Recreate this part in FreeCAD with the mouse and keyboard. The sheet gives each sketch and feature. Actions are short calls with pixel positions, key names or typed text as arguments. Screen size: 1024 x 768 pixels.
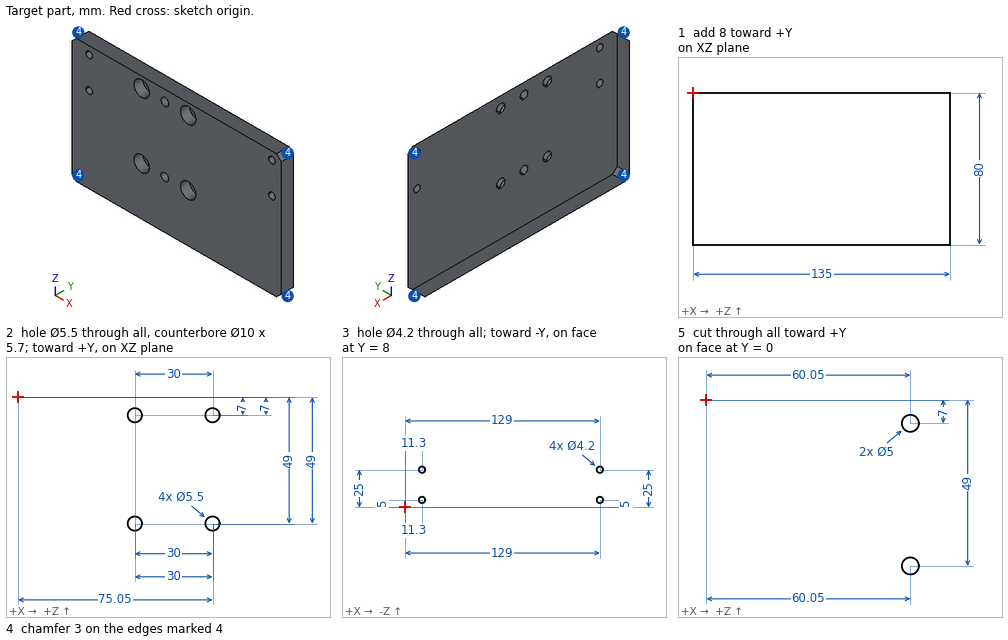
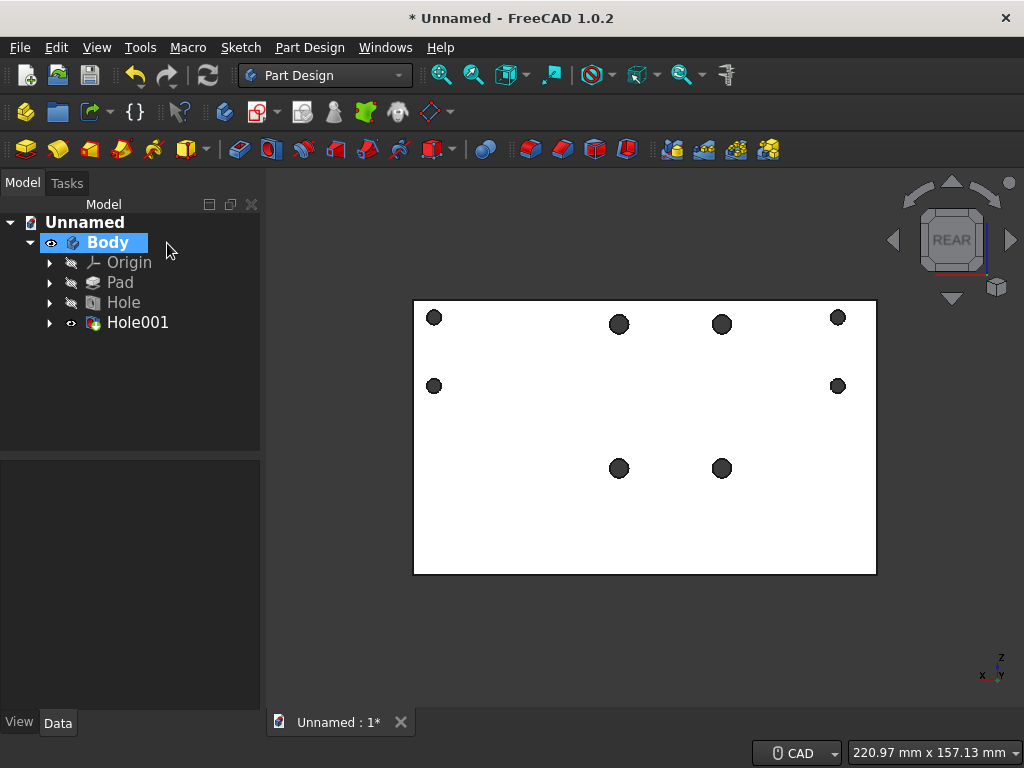
key(0)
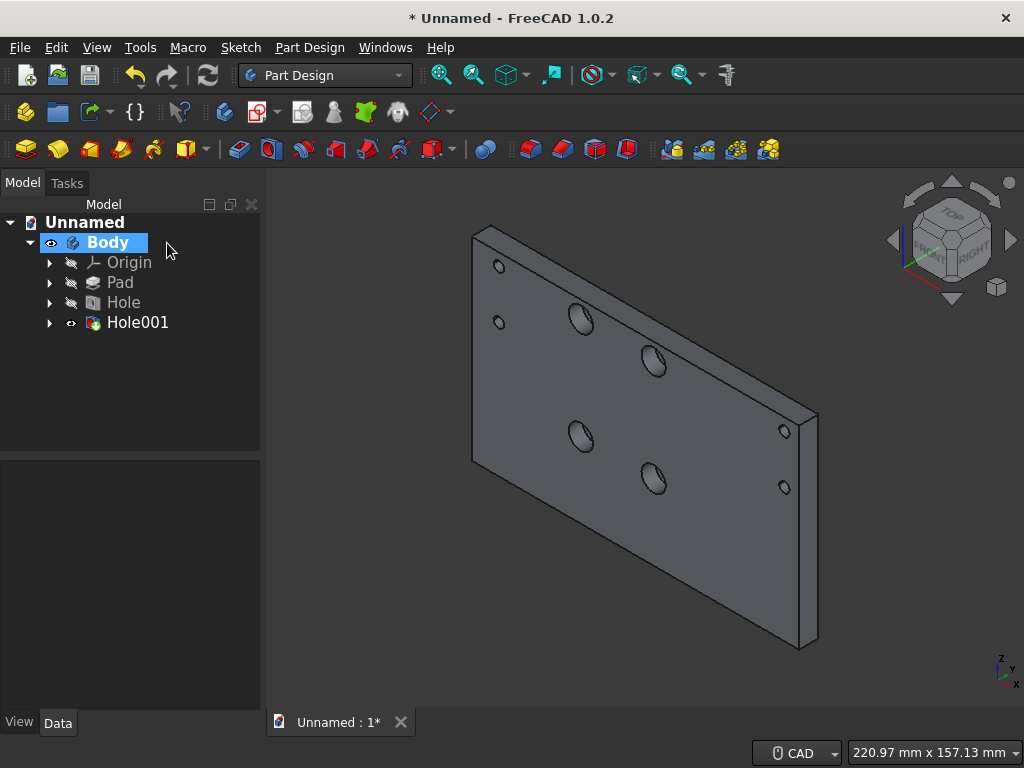
click(809, 419)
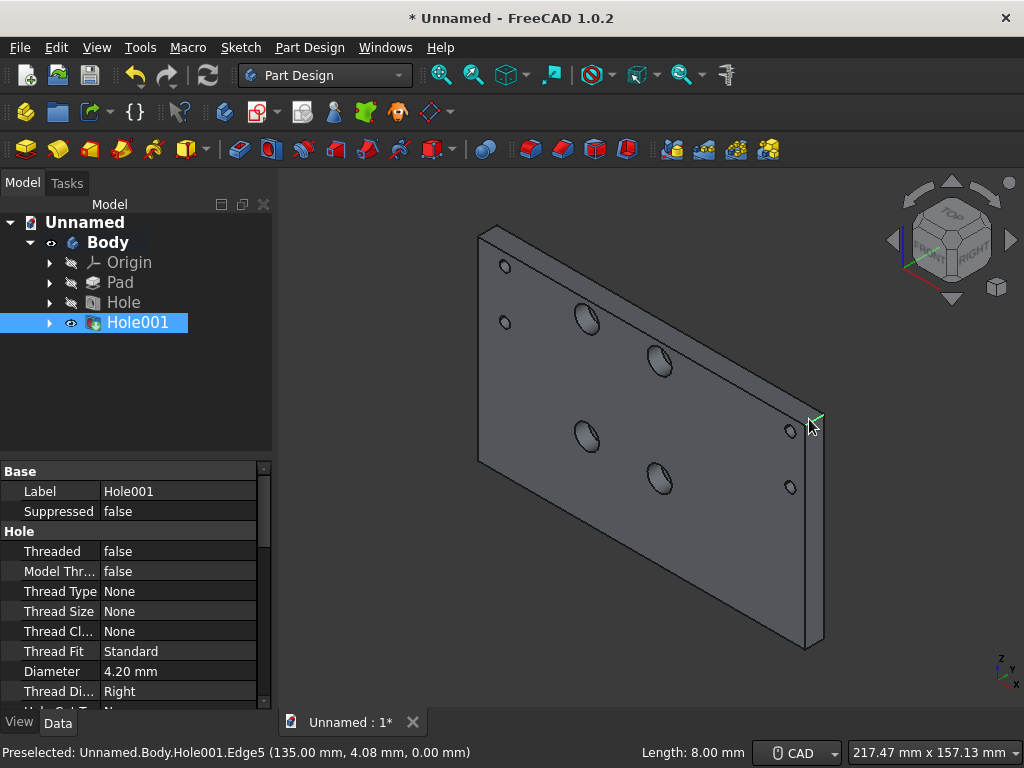
key(2)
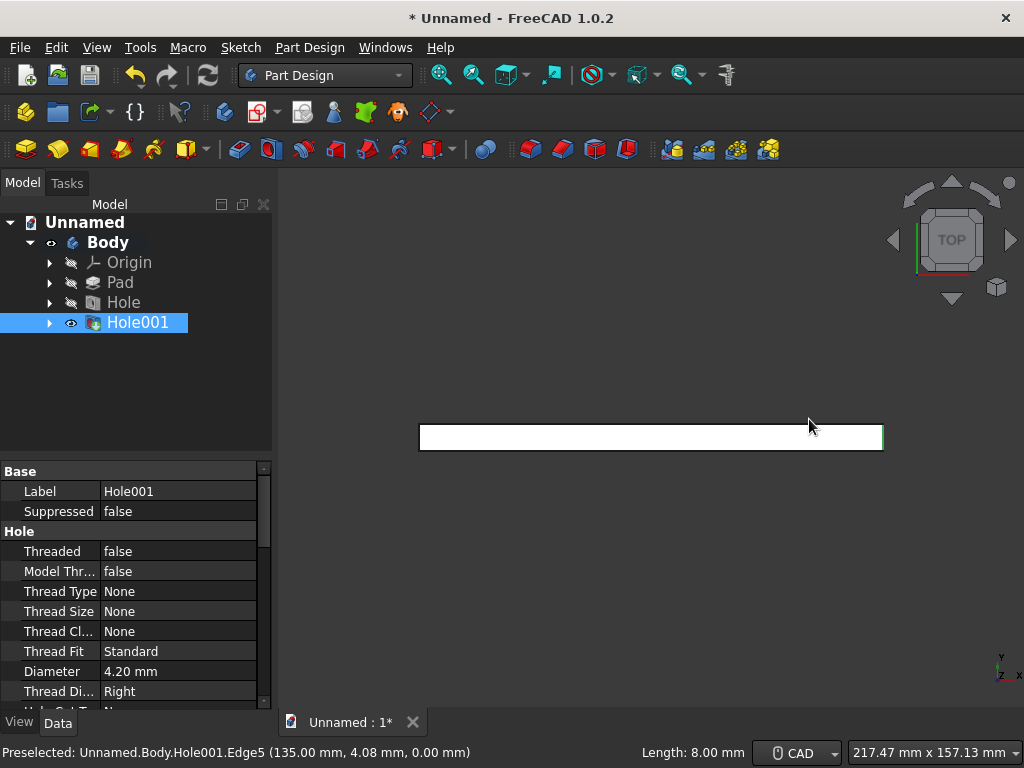
click(419, 437, ctrl)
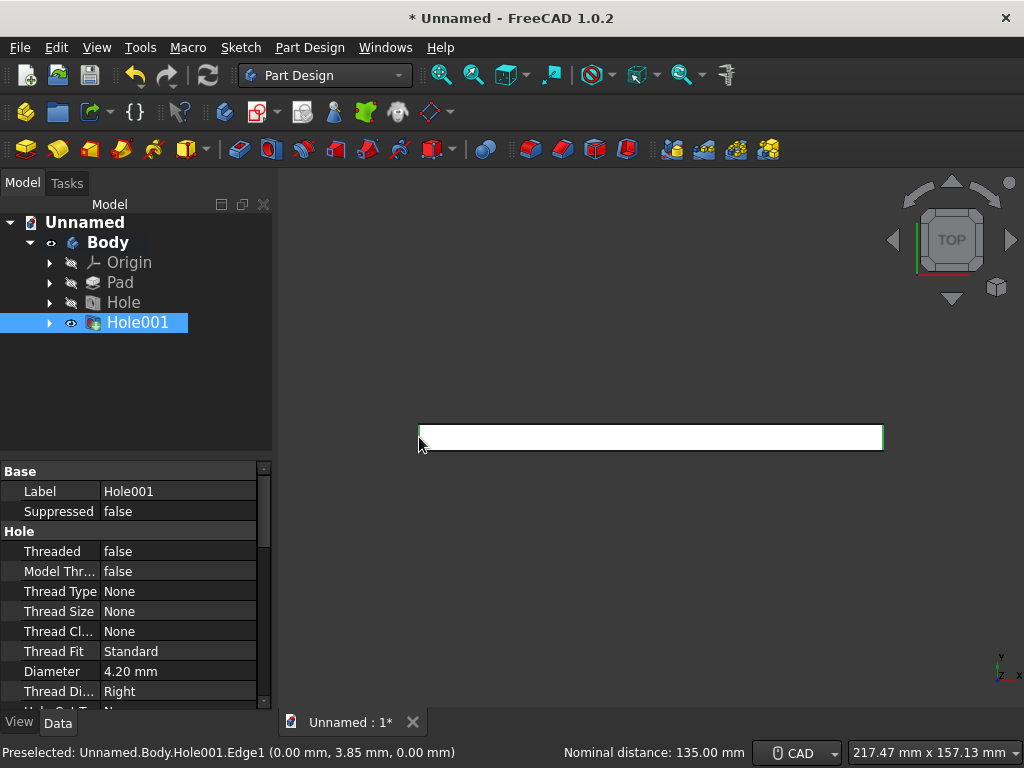
key(1)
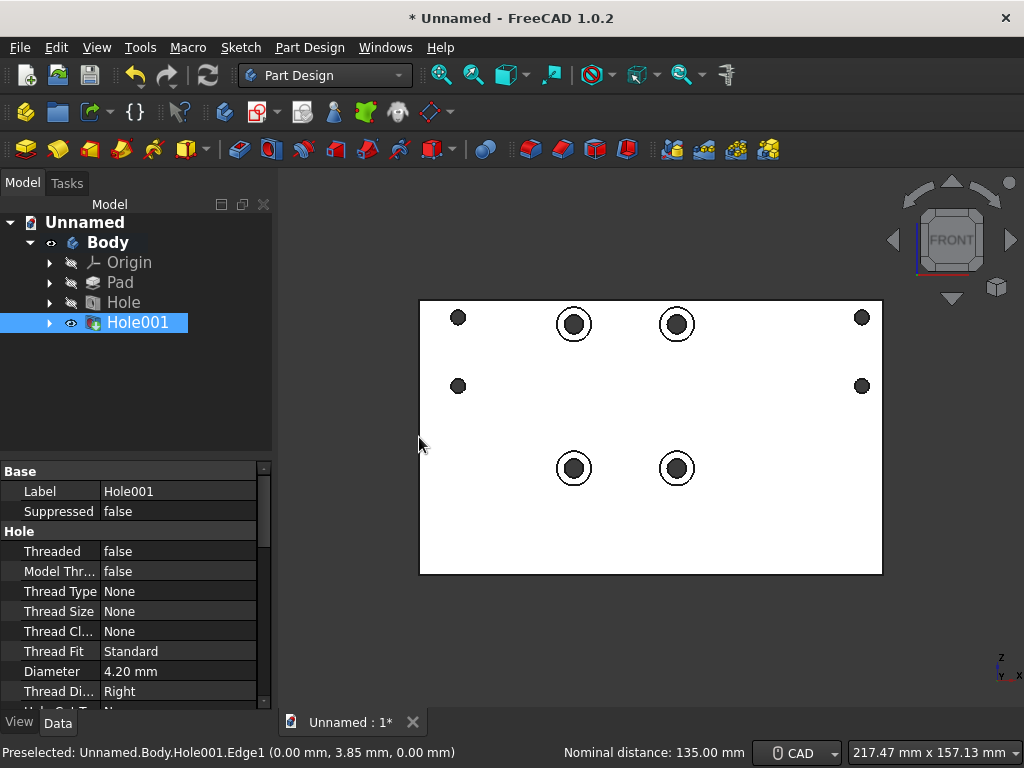
key(3)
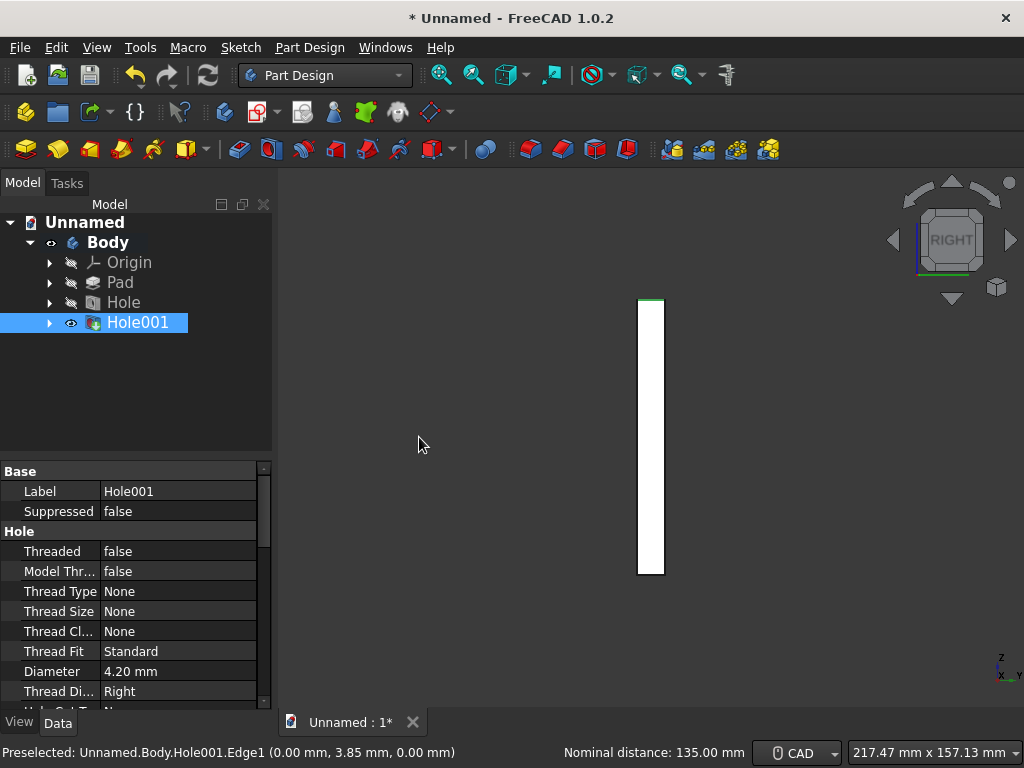
click(651, 574, ctrl)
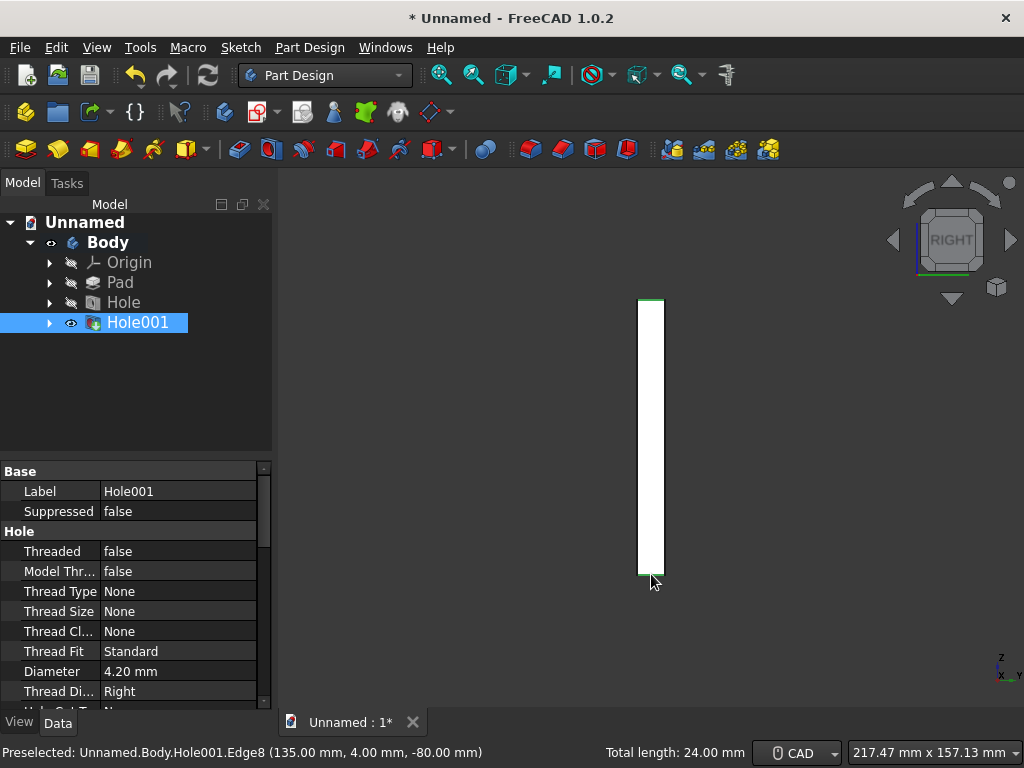
key(5)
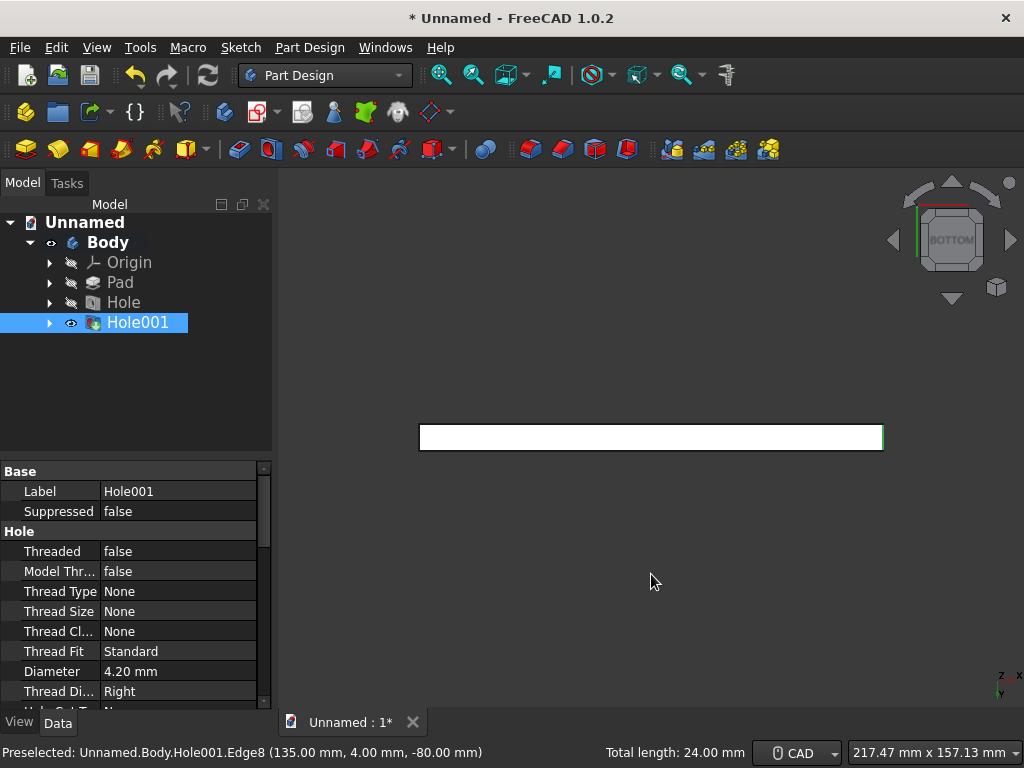
click(419, 437, ctrl)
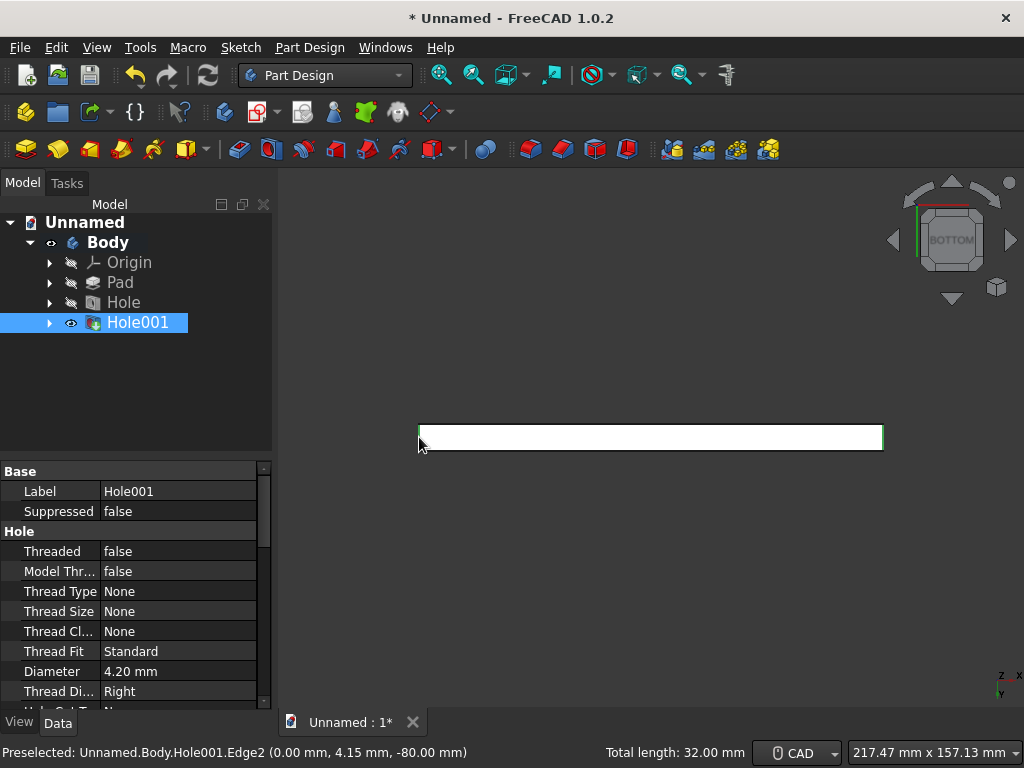
click(564, 150)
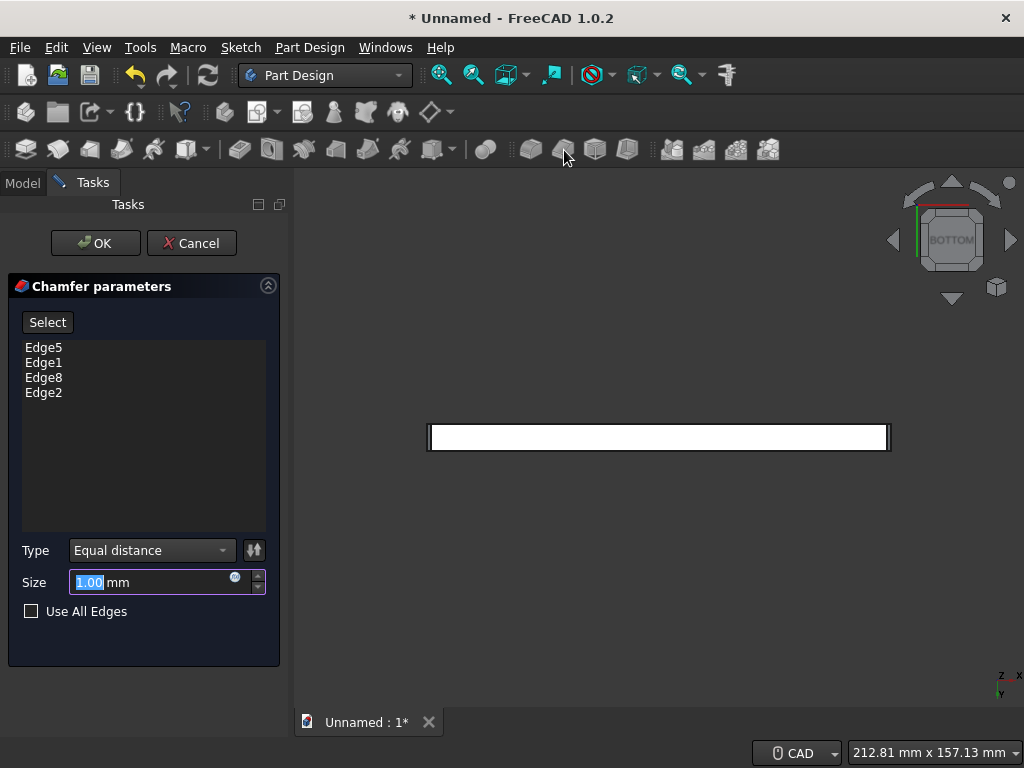
text(3)
key(Tab)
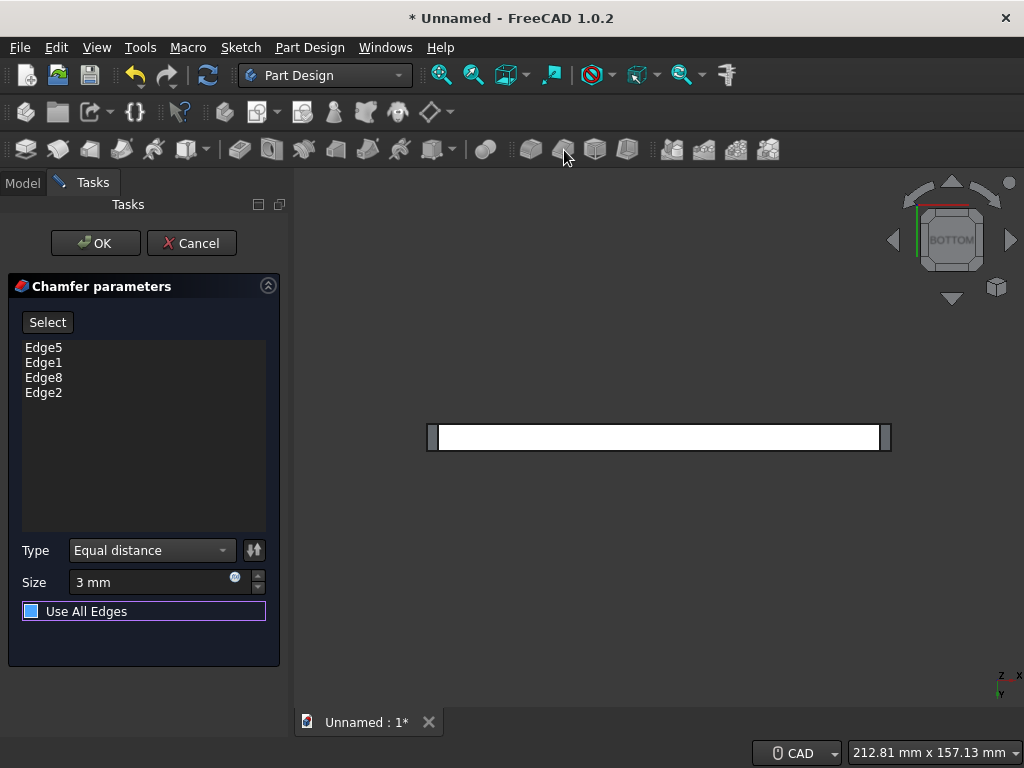
click(96, 243)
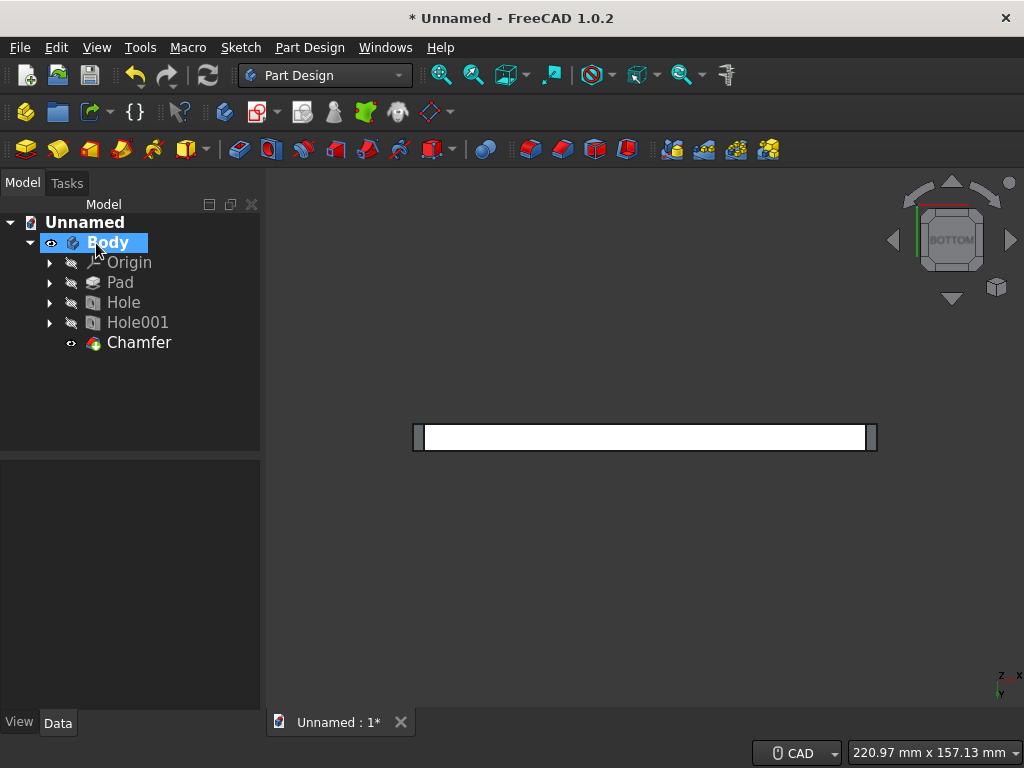
key(0)